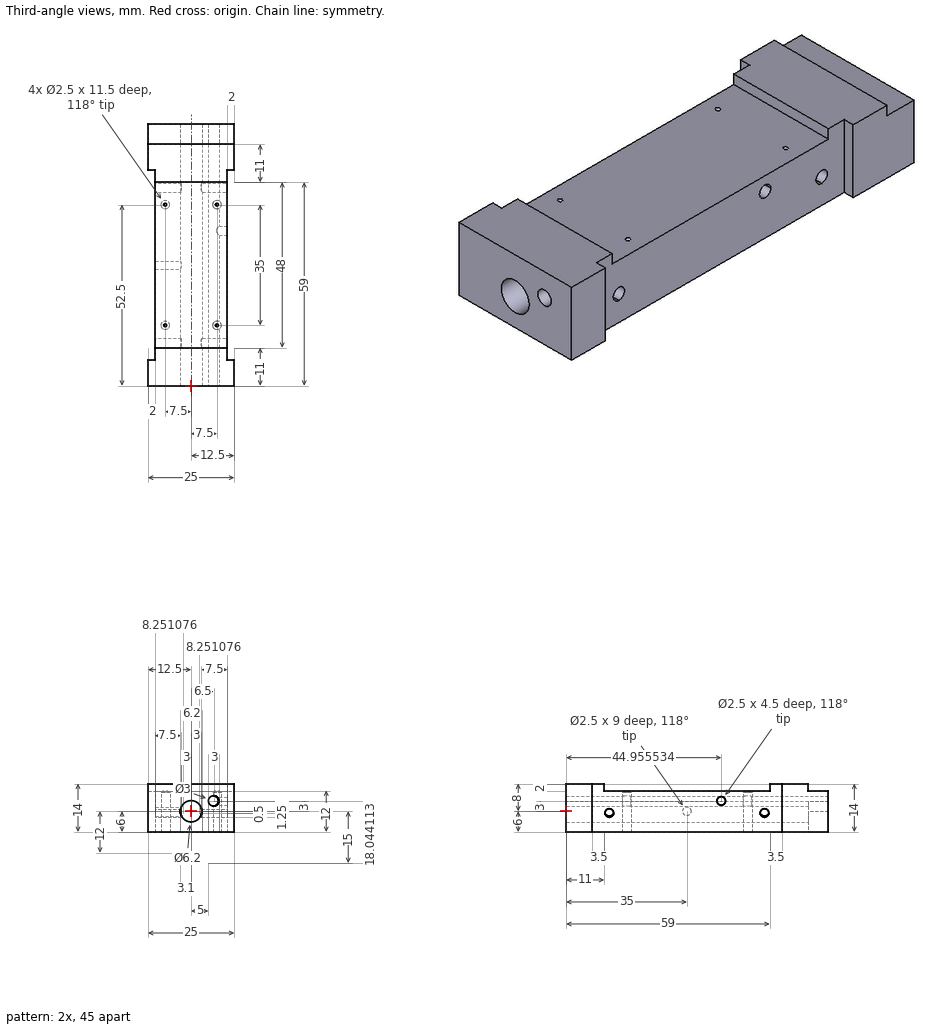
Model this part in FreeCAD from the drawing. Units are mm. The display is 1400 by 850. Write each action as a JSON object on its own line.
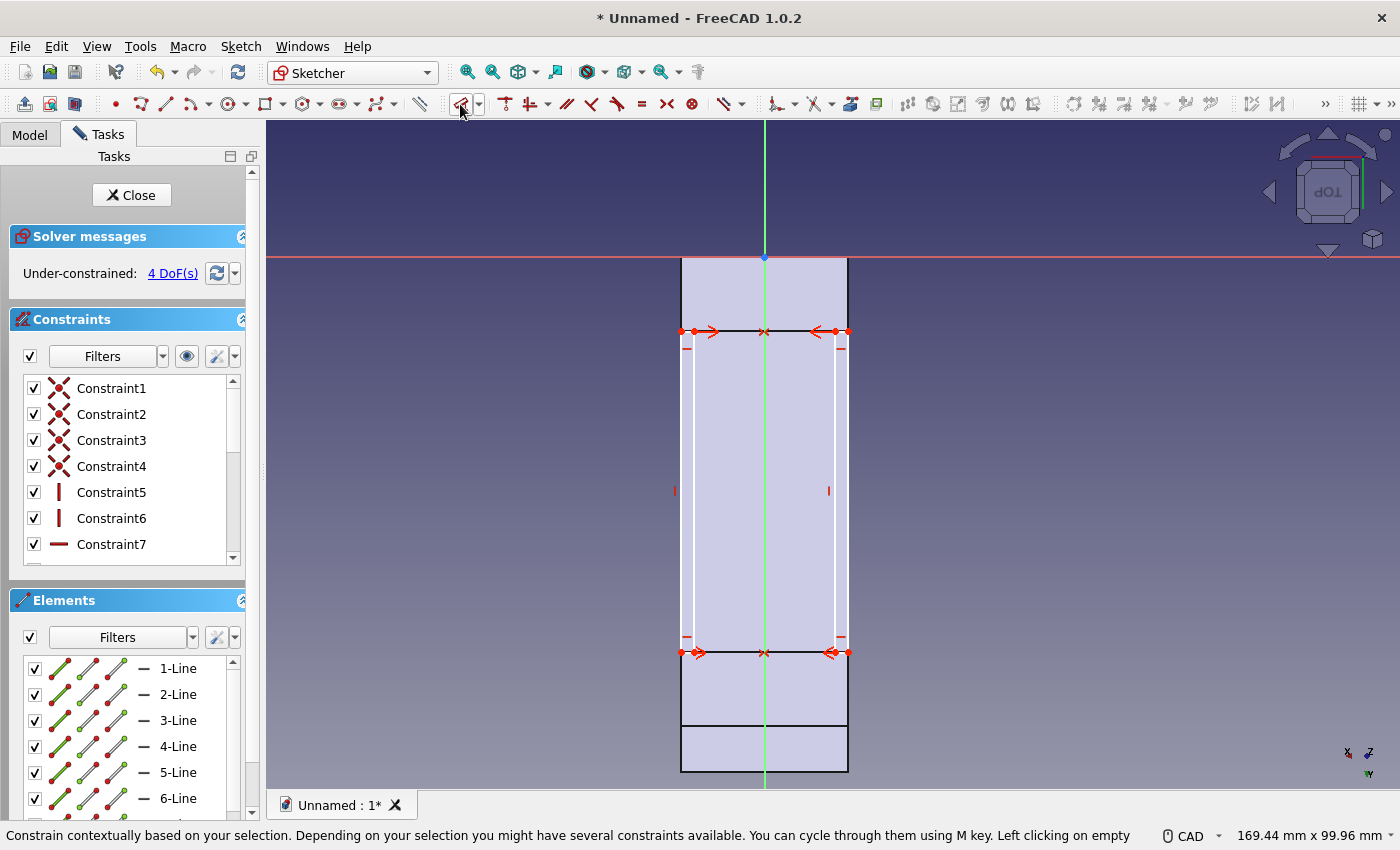
{"action": "scroll", "coordinate": [688, 653], "scroll_direction": "up", "scroll_amount": 6}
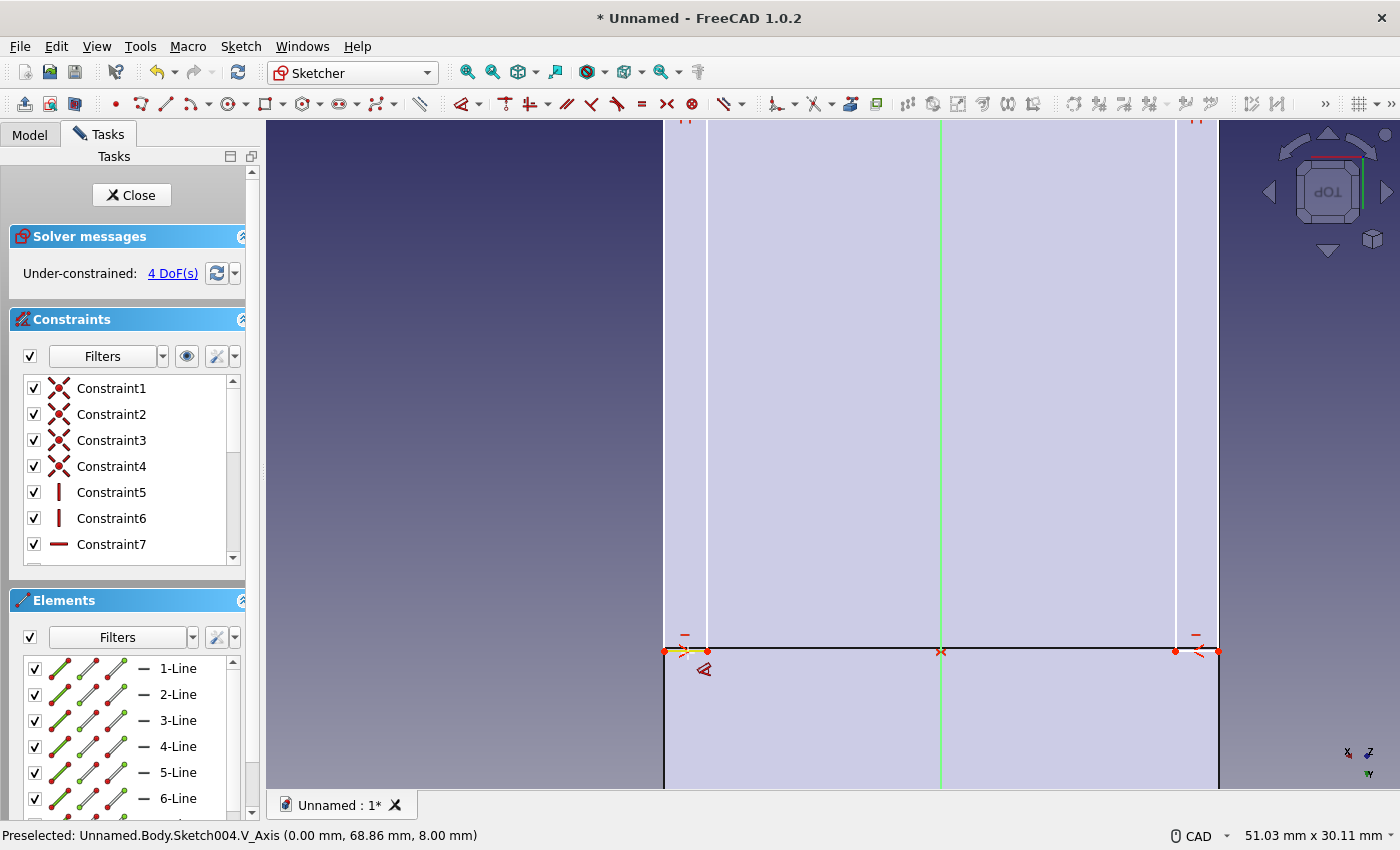
{"action": "left_click", "coordinate": [686, 651]}
{"action": "left_click", "coordinate": [686, 685]}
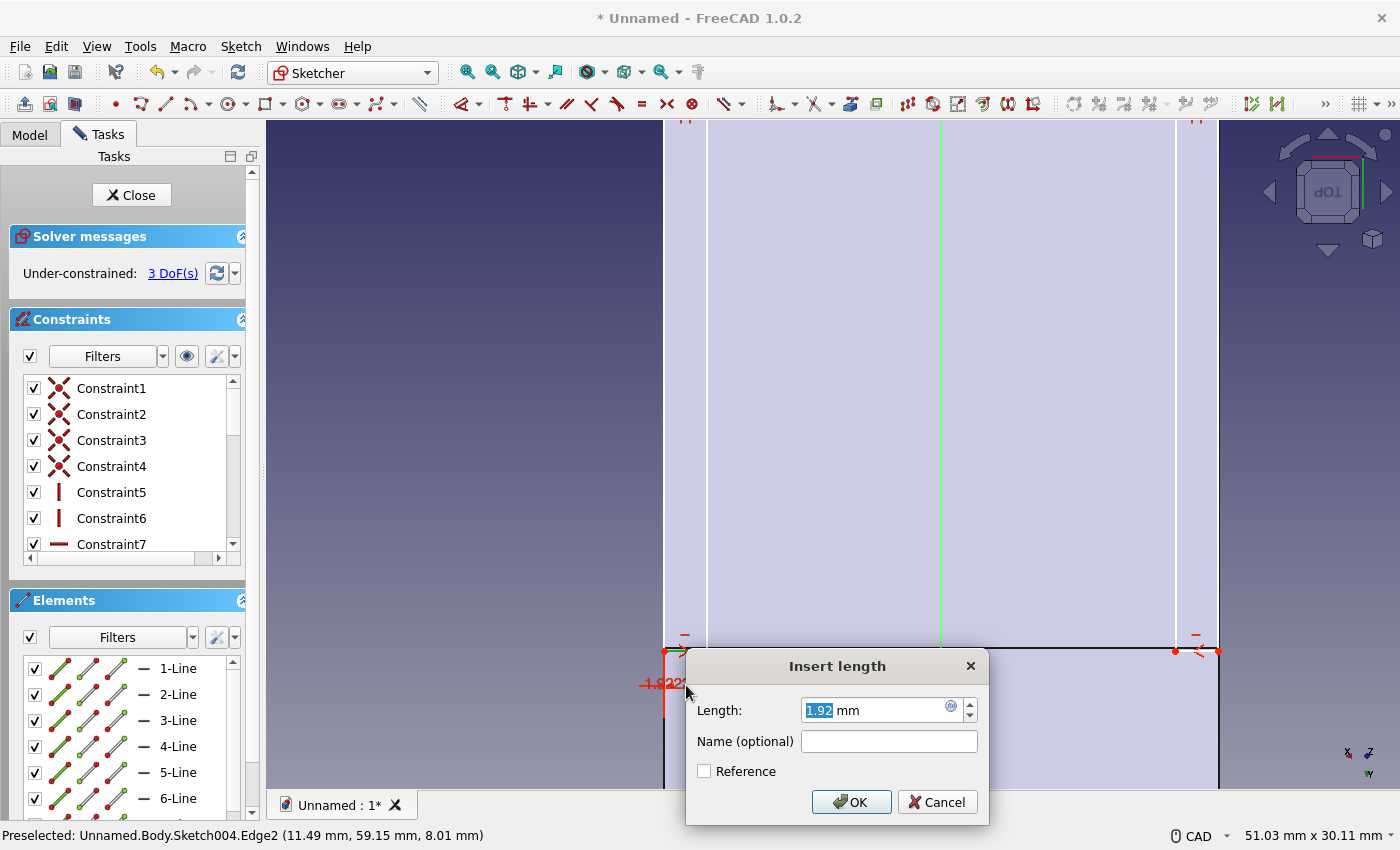
{"action": "type", "text": "2"}
{"action": "key", "text": "Return"}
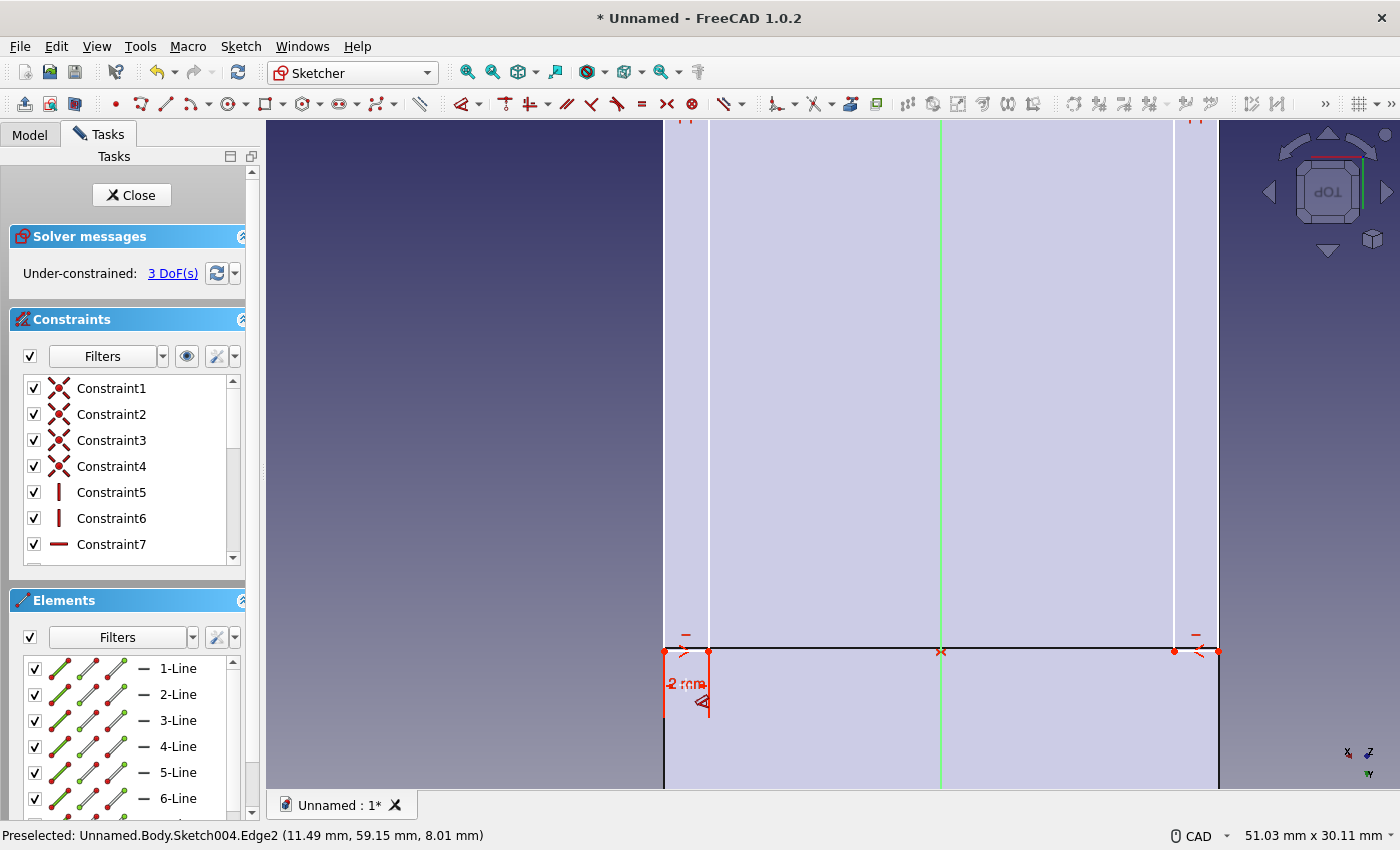
{"action": "left_click", "coordinate": [664, 331]}
{"action": "left_click", "coordinate": [630, 400]}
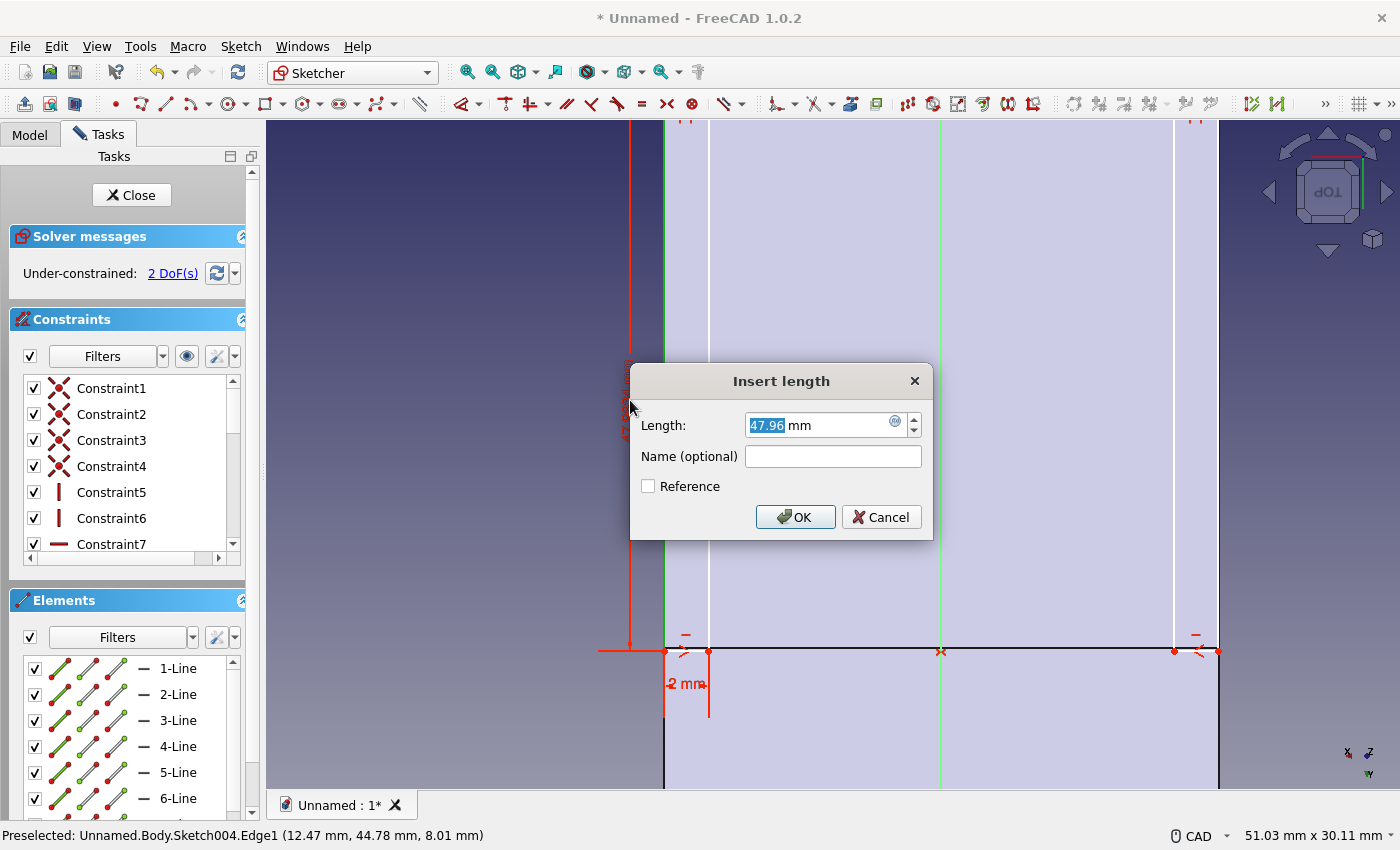
{"action": "type", "text": "48"}
{"action": "key", "text": "Return"}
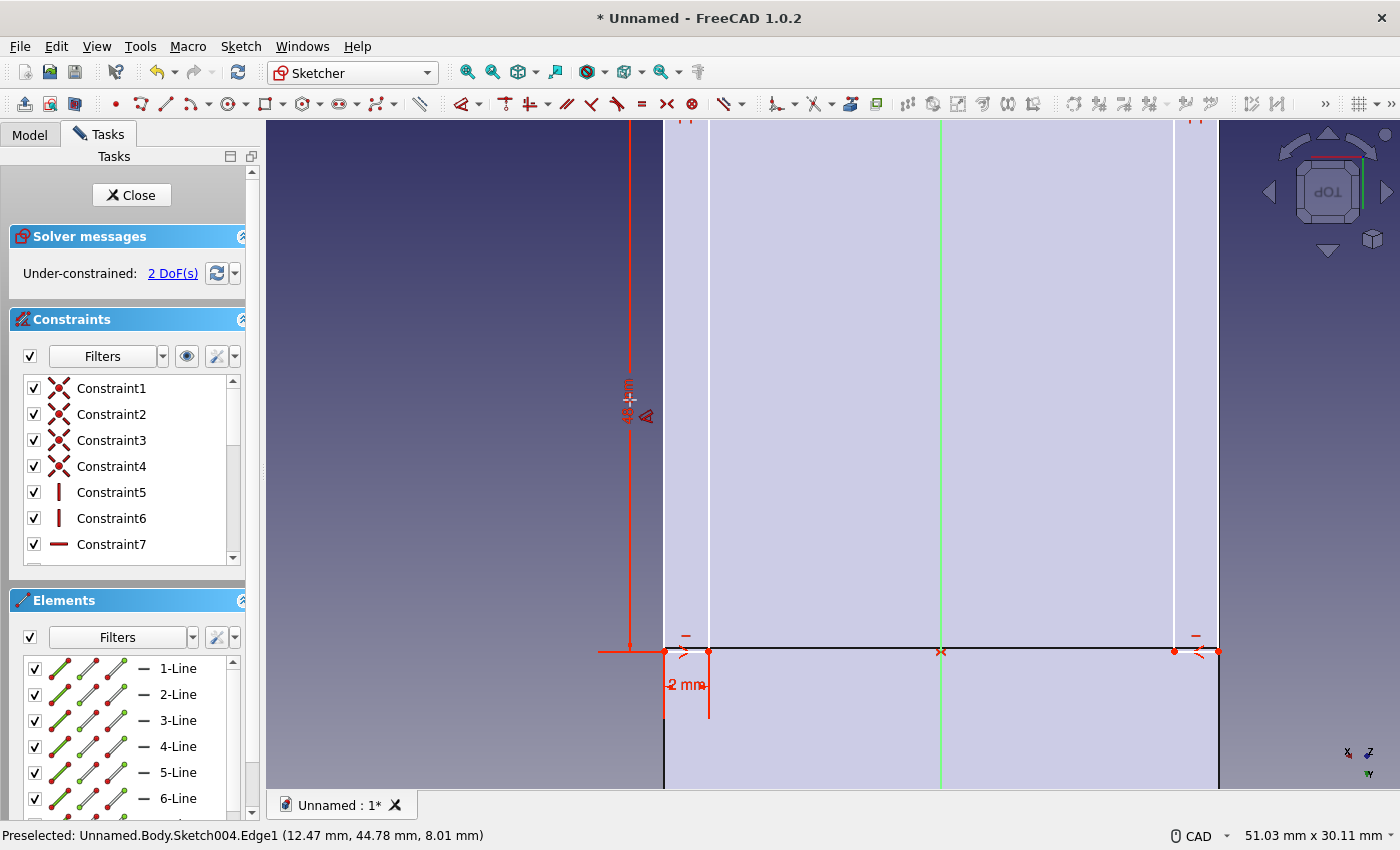
{"action": "scroll", "coordinate": [688, 654], "scroll_direction": "down", "scroll_amount": 6}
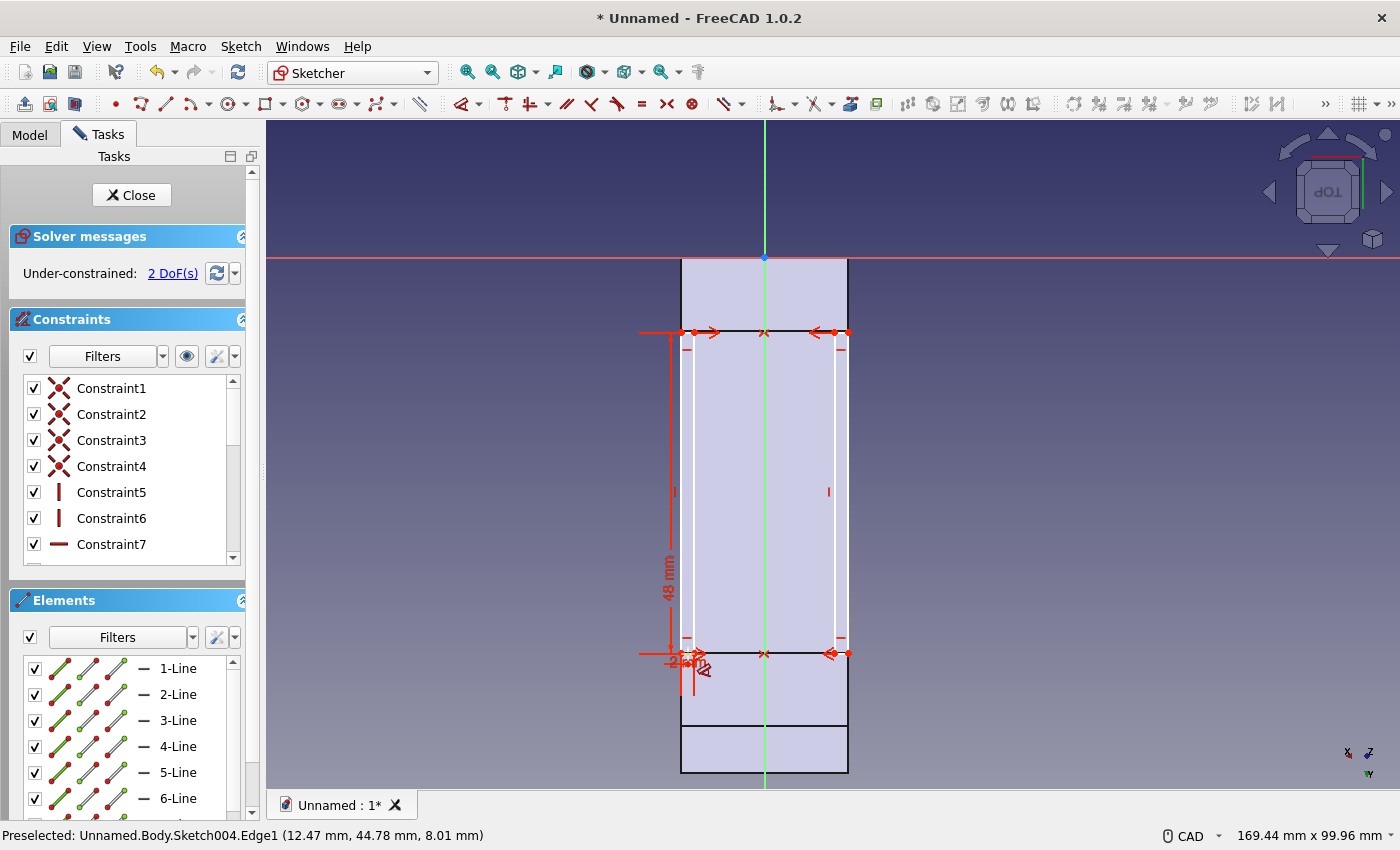
{"action": "left_click", "coordinate": [681, 333]}
{"action": "left_click", "coordinate": [647, 295]}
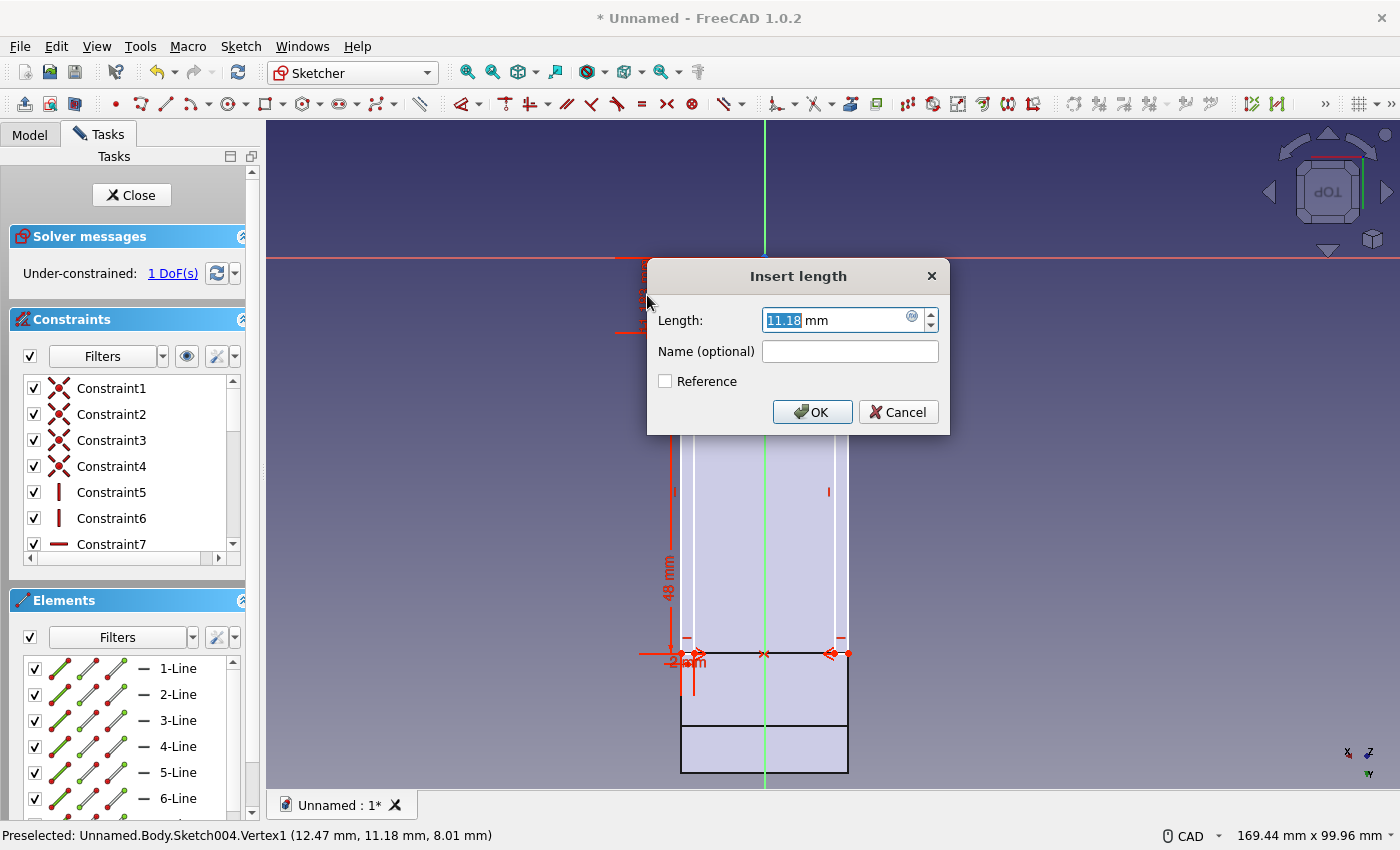
{"action": "type", "text": "11"}
{"action": "key", "text": "Return"}